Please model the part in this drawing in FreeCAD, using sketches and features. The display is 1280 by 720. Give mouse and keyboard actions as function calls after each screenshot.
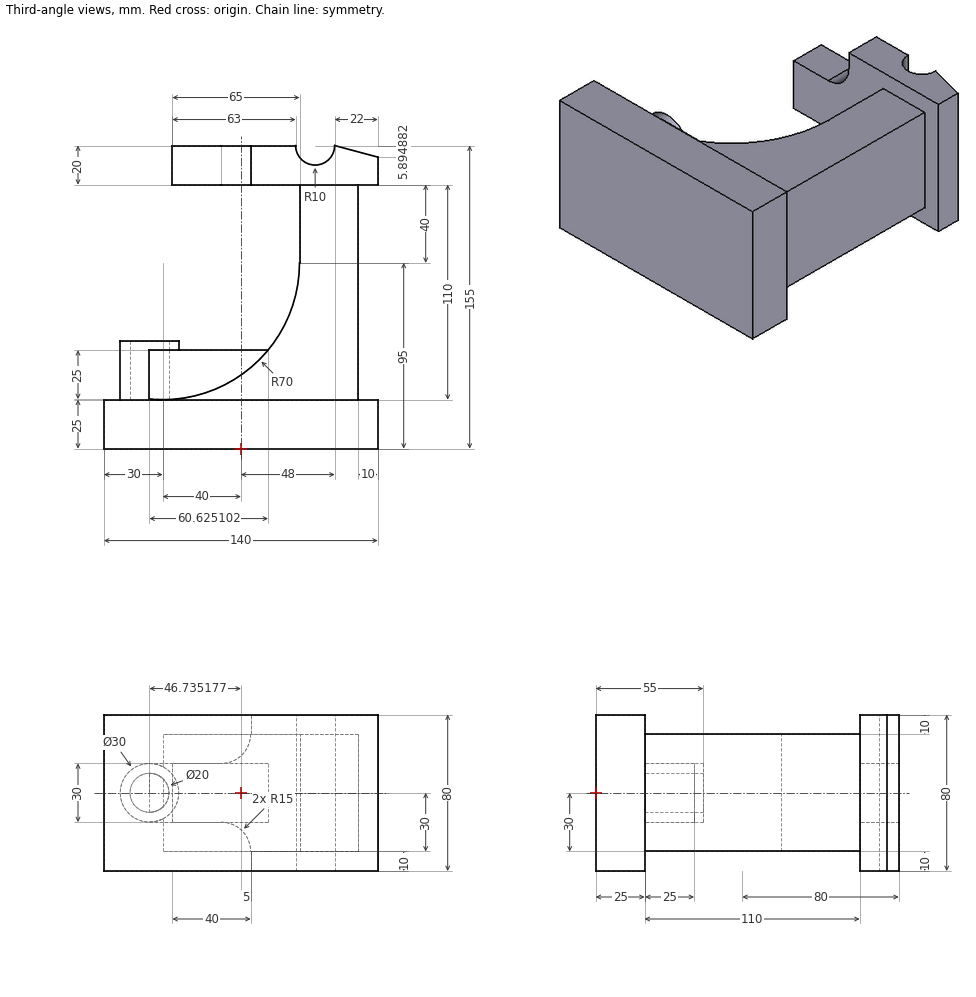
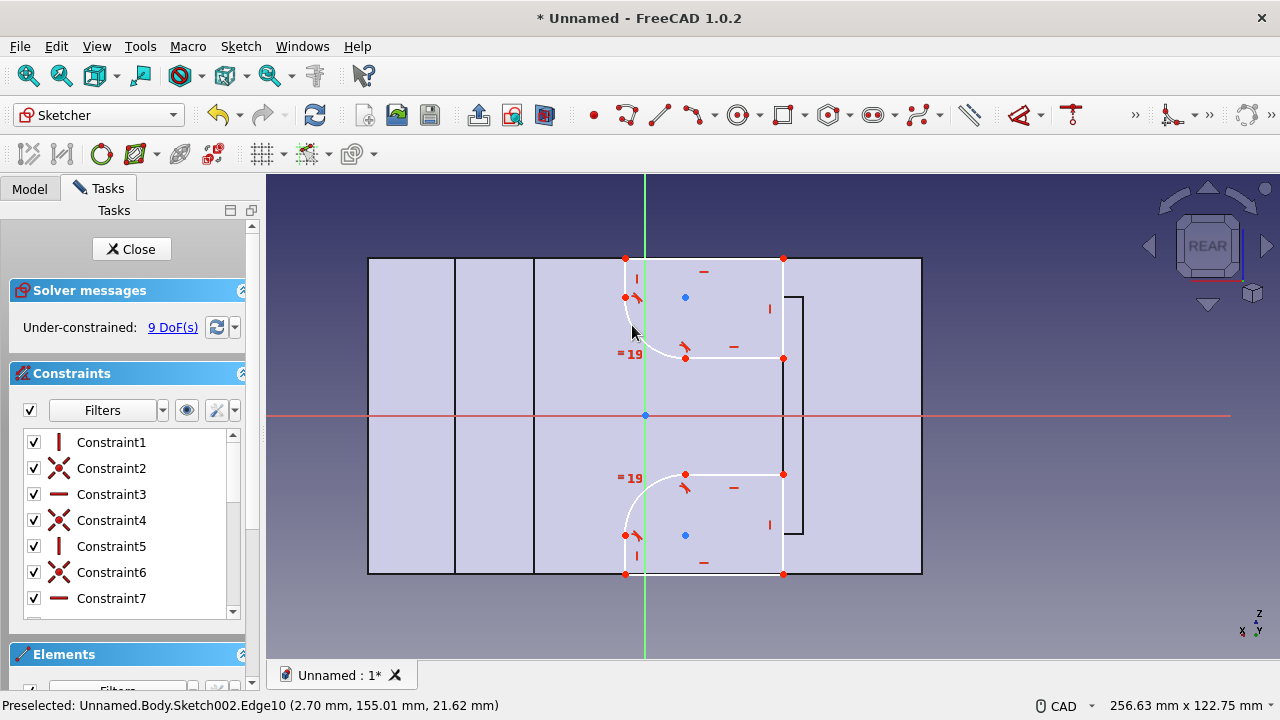
click(685, 535)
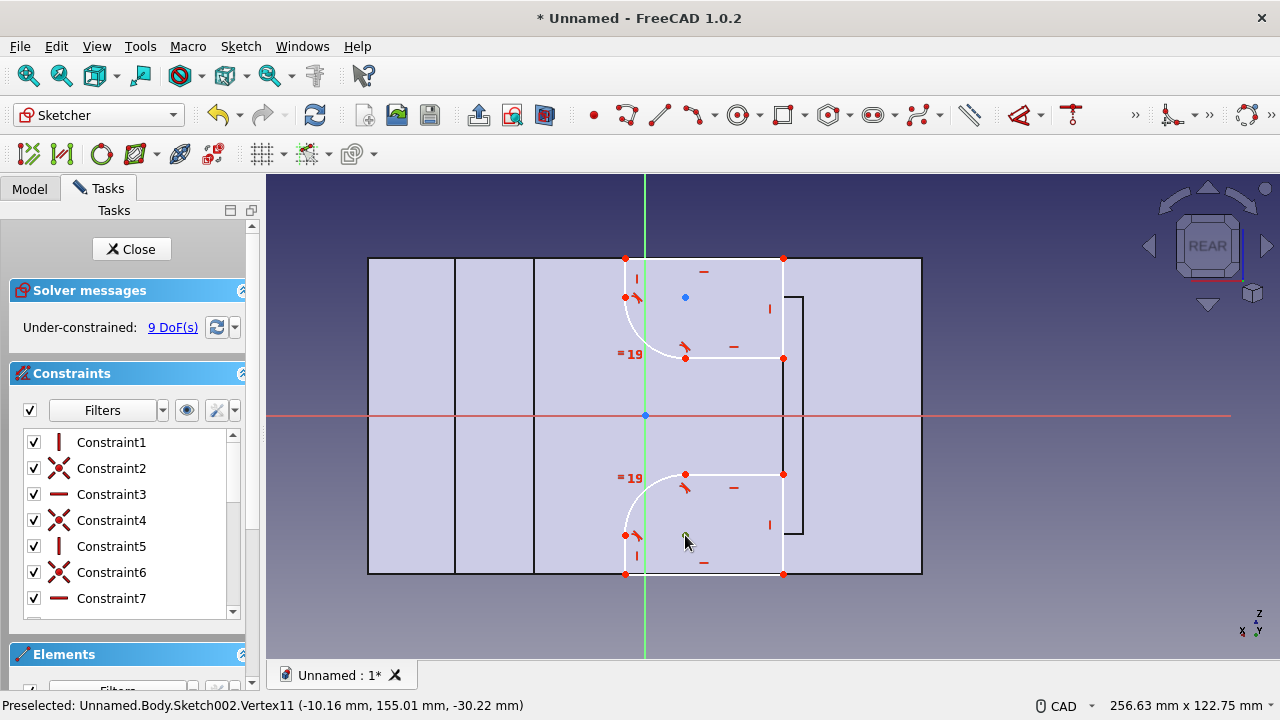
click(685, 298)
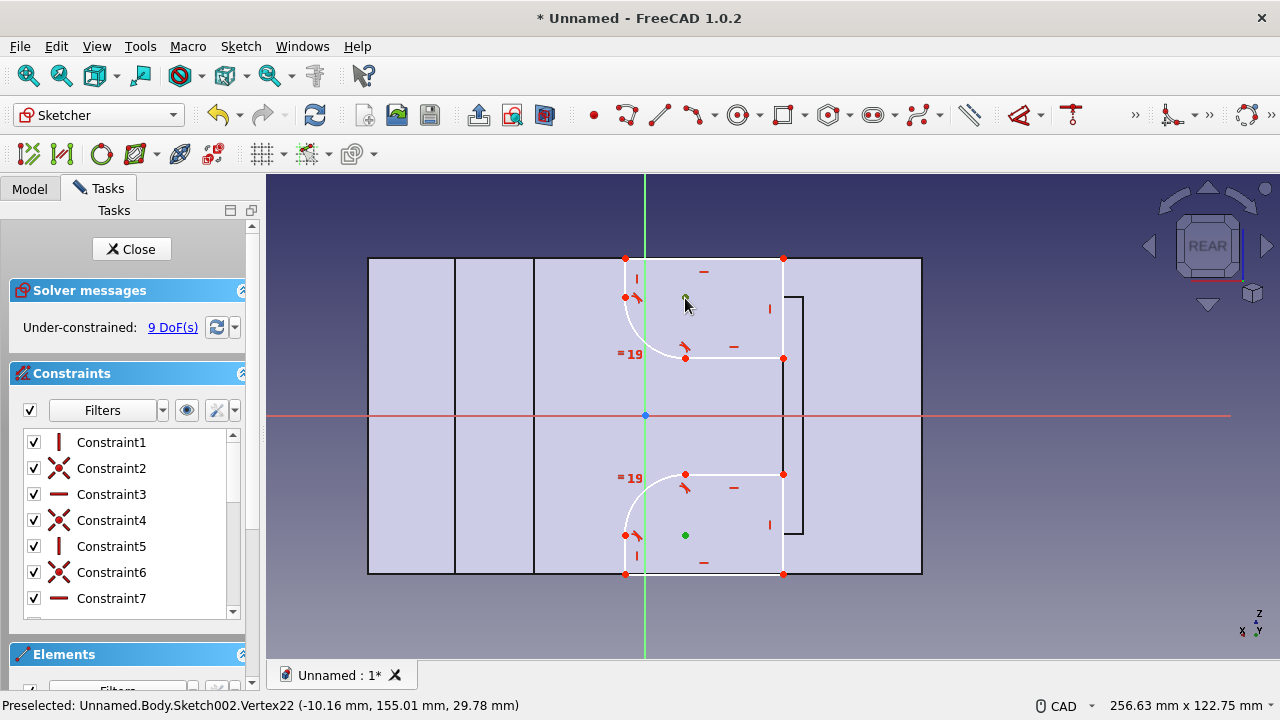
click(353, 416)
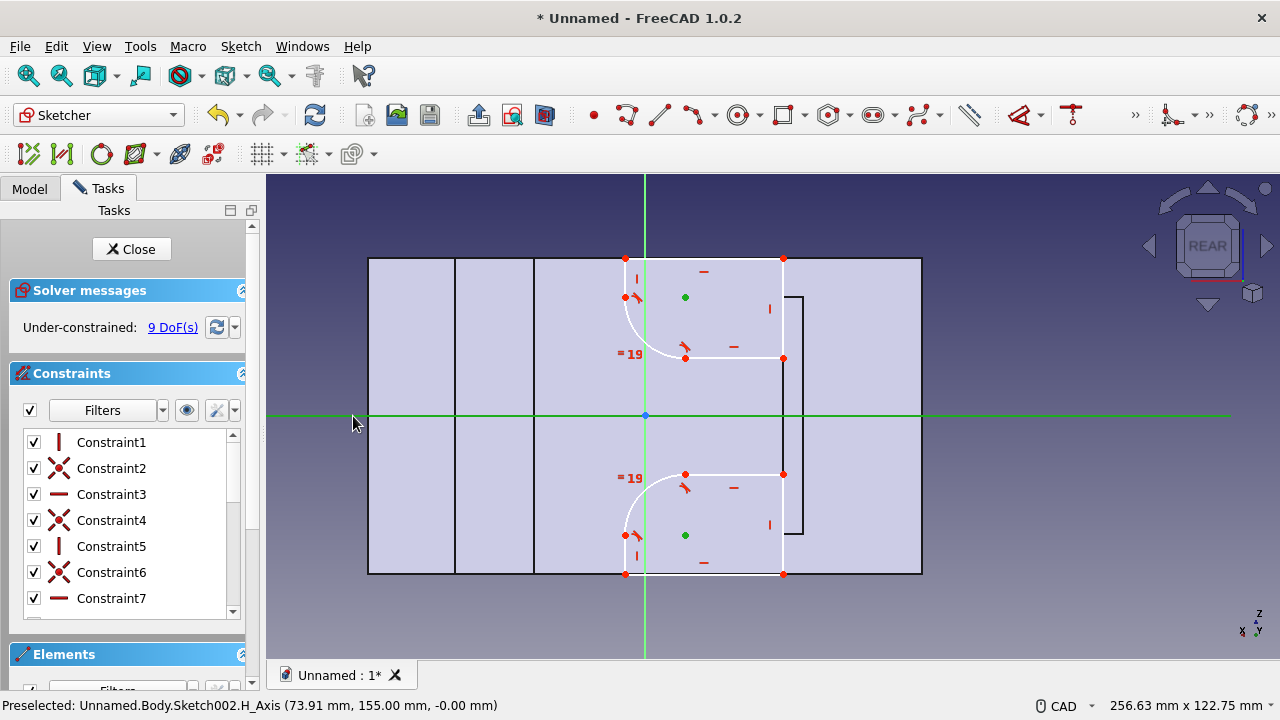
key(s)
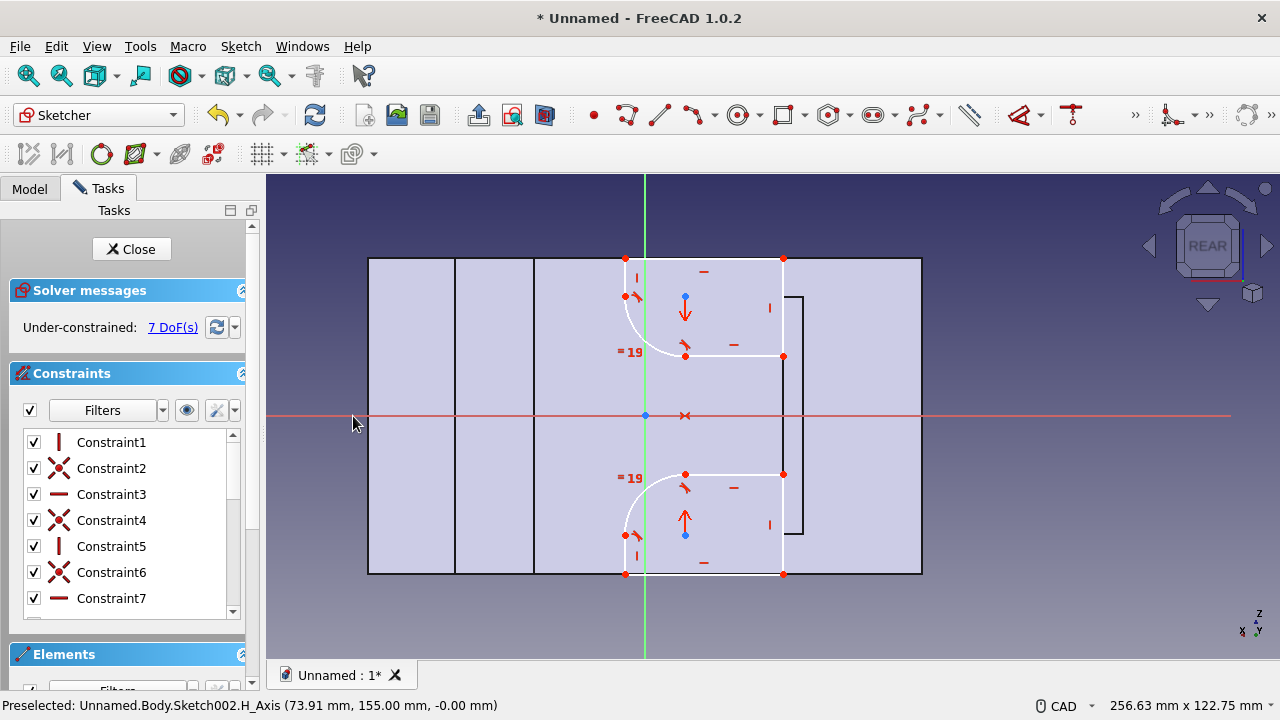
click(783, 575)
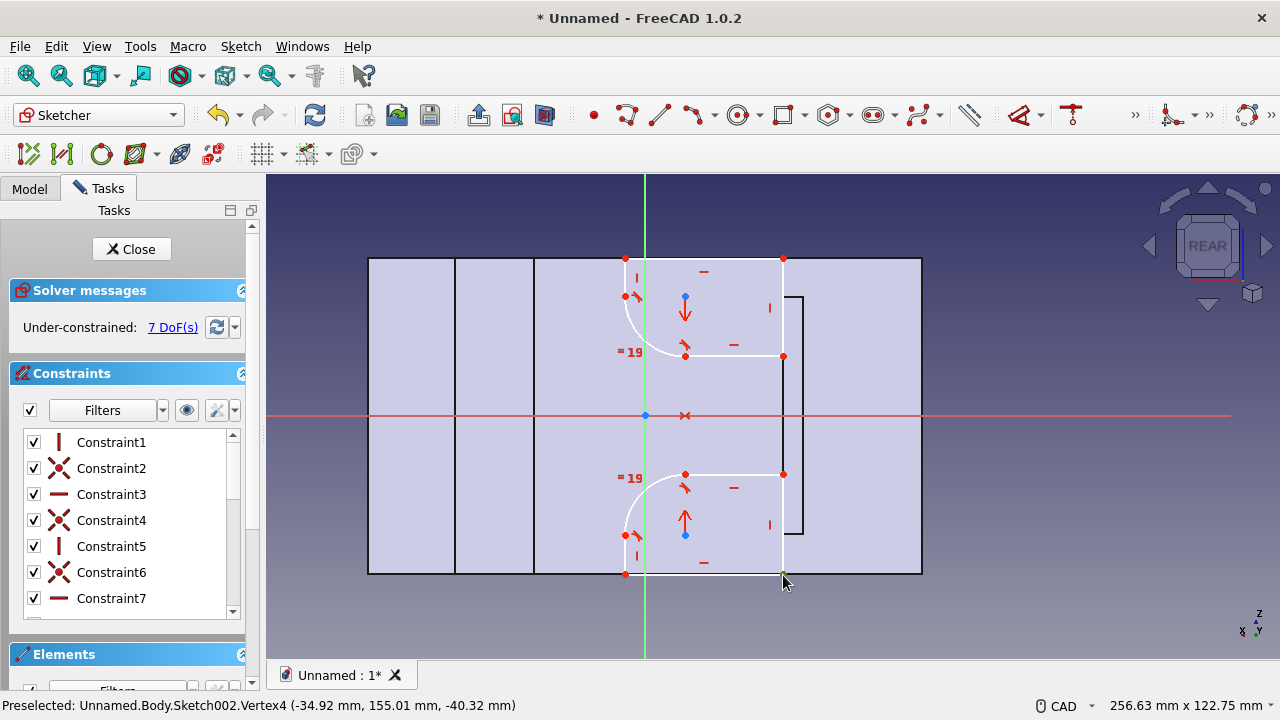
click(783, 259)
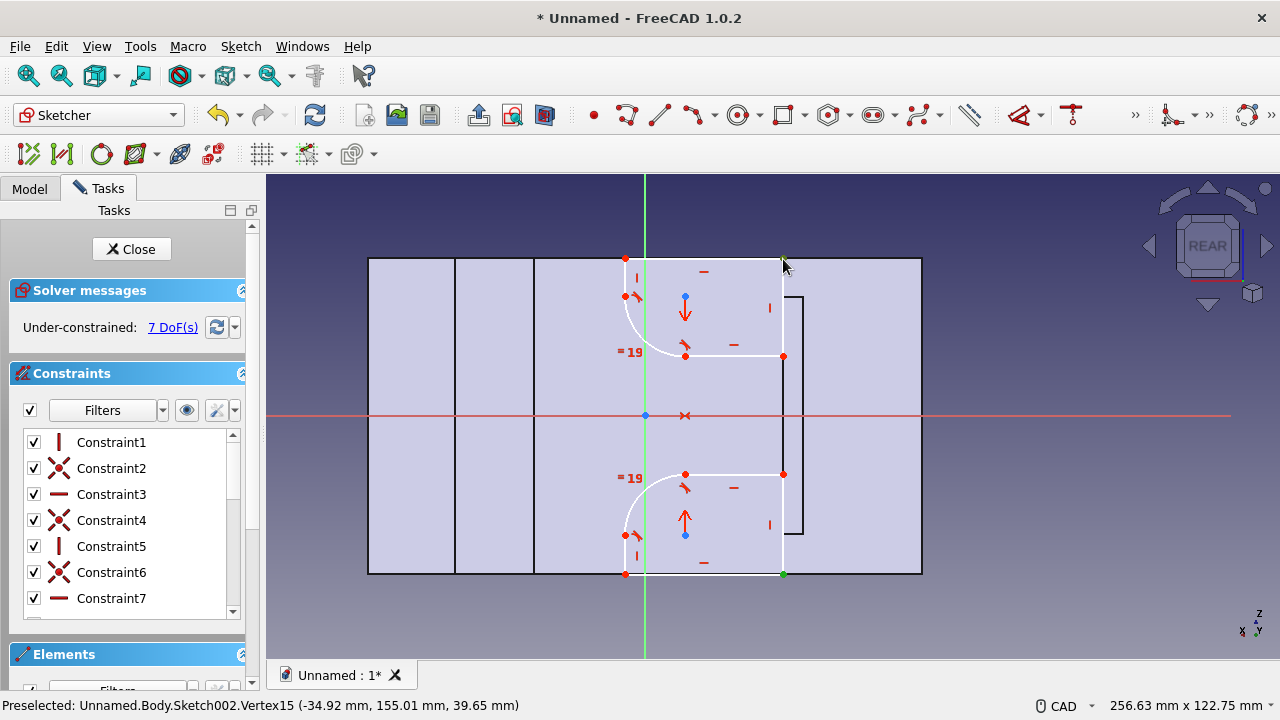
click(353, 416)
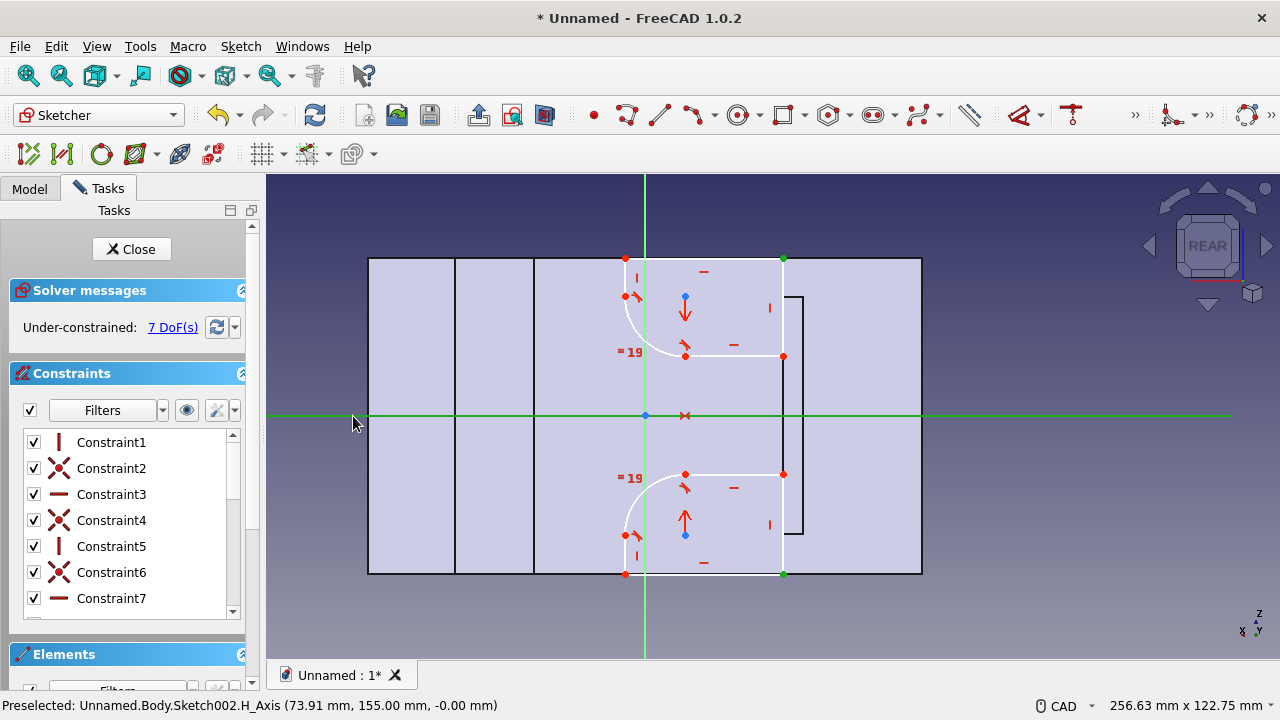
key(s)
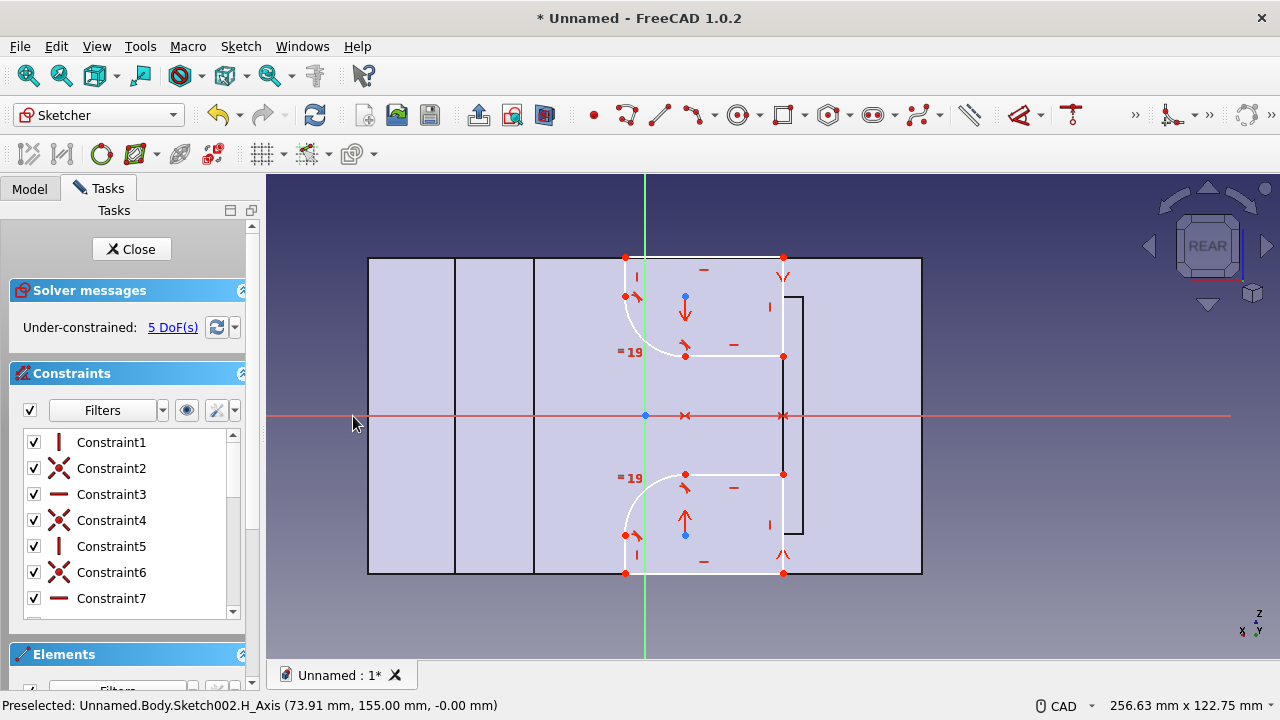
click(1018, 116)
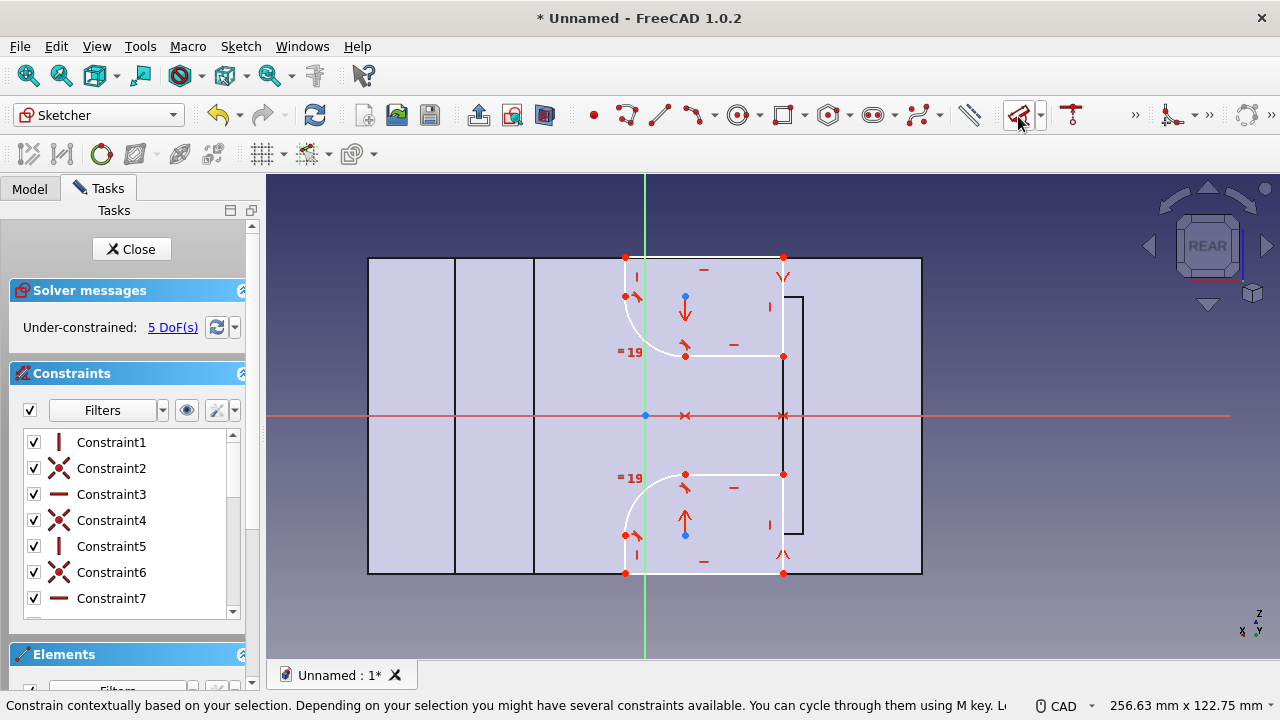
click(658, 481)
click(688, 443)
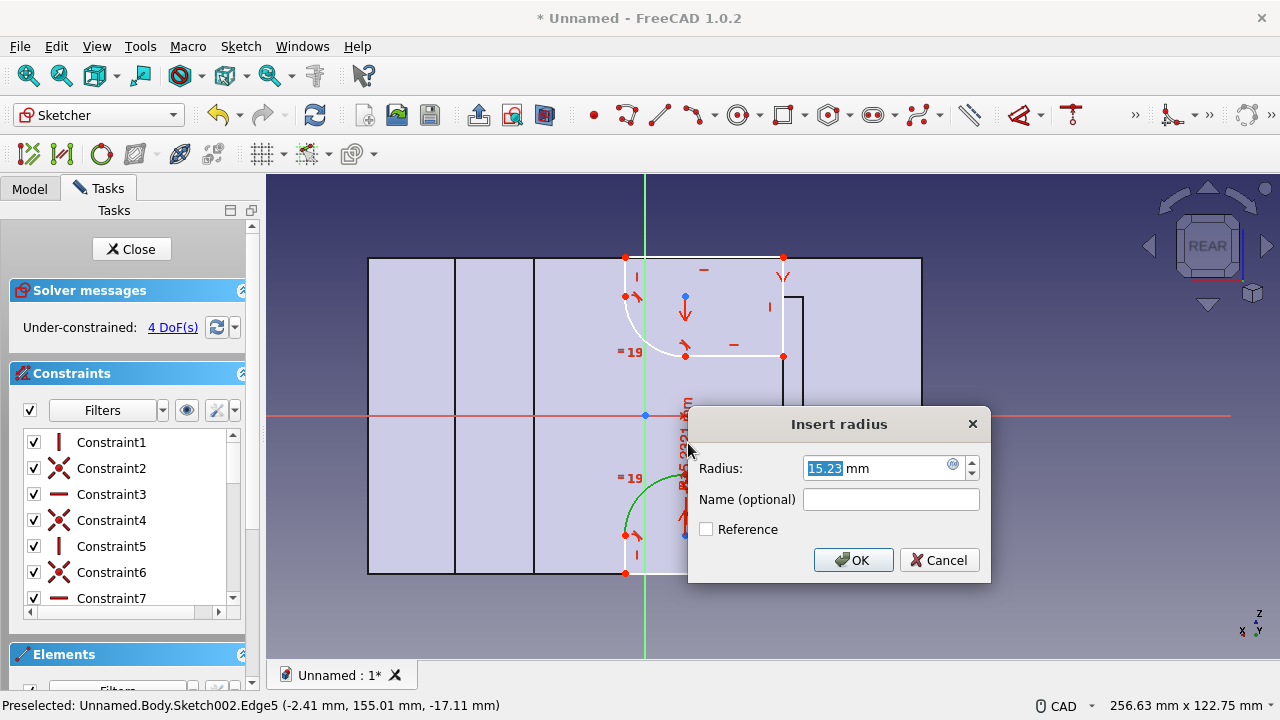
text(15)
key(Return)